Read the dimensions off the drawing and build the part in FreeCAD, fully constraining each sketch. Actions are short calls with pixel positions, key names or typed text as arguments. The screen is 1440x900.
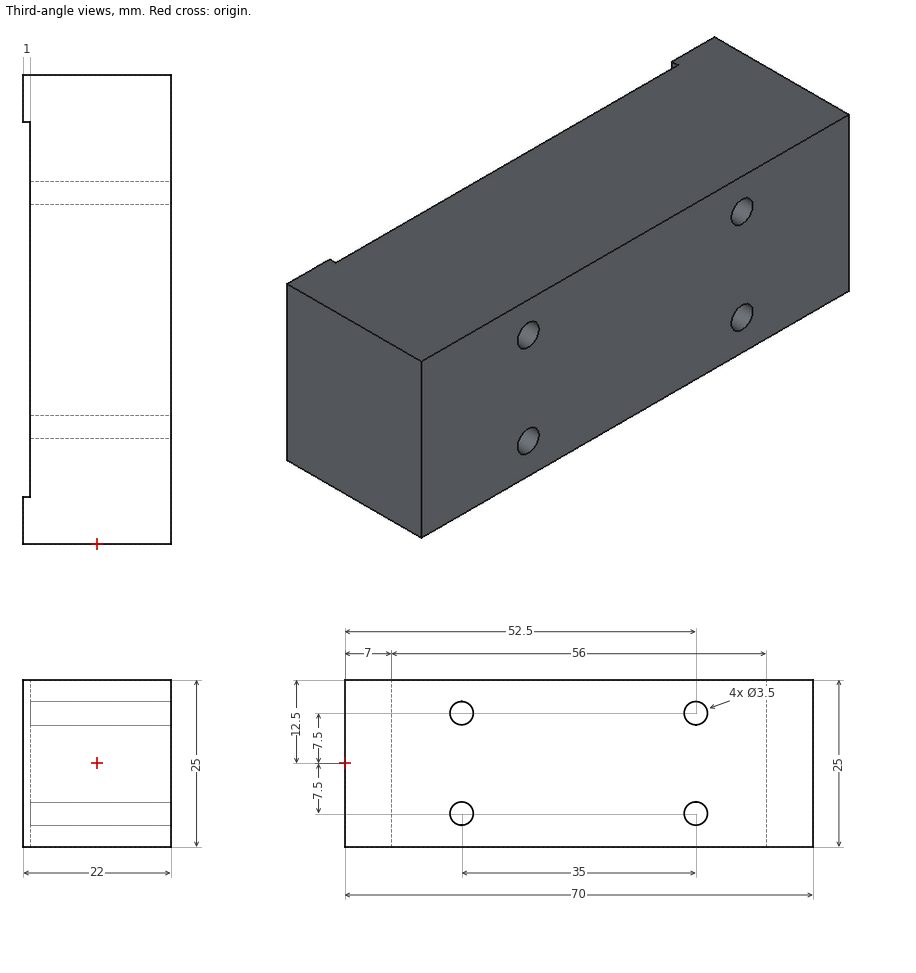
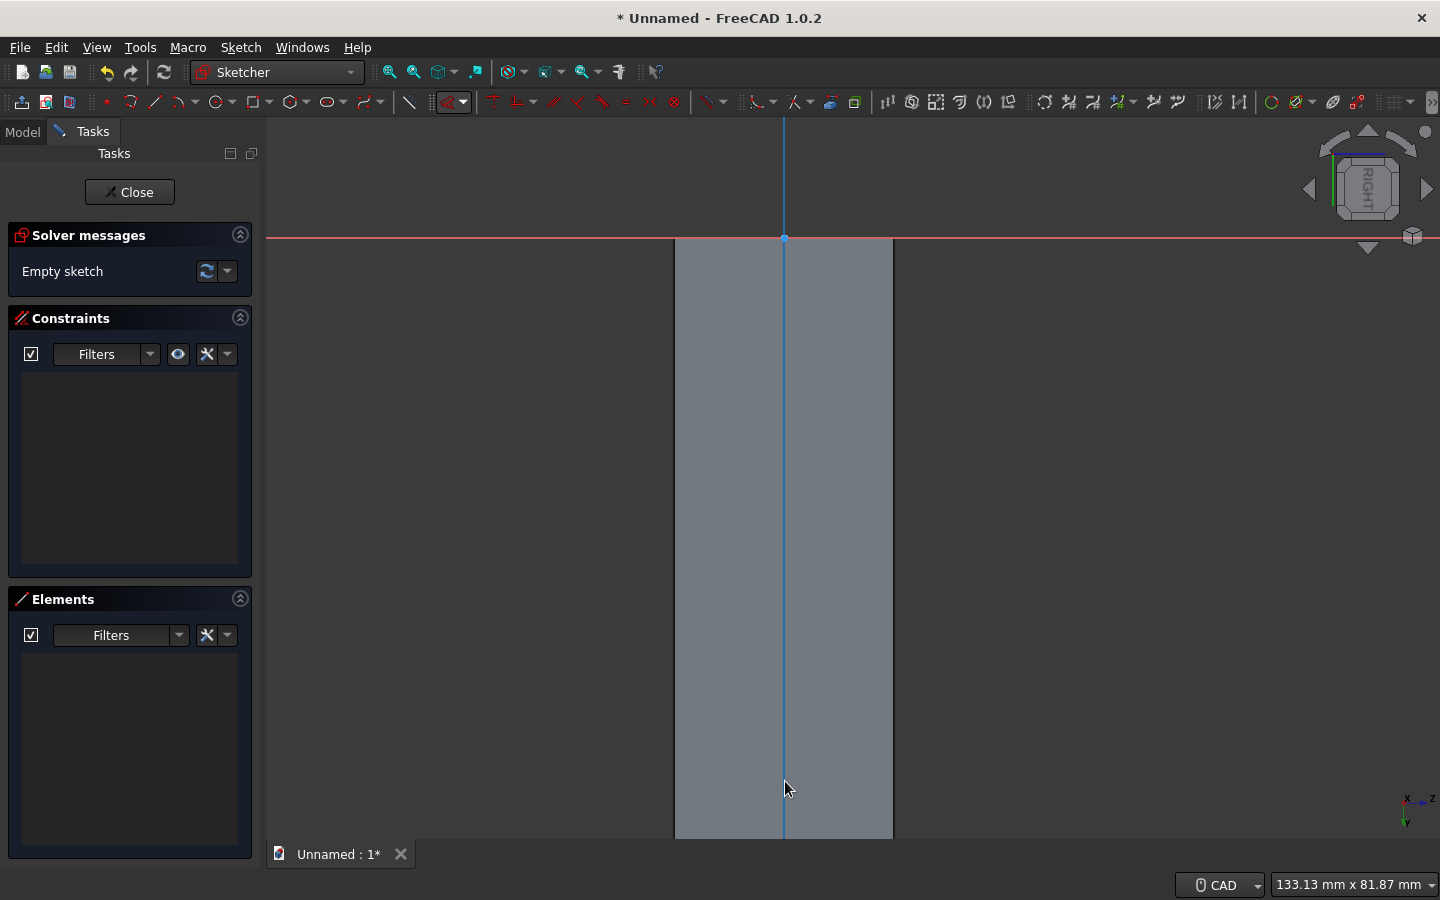
click(216, 102)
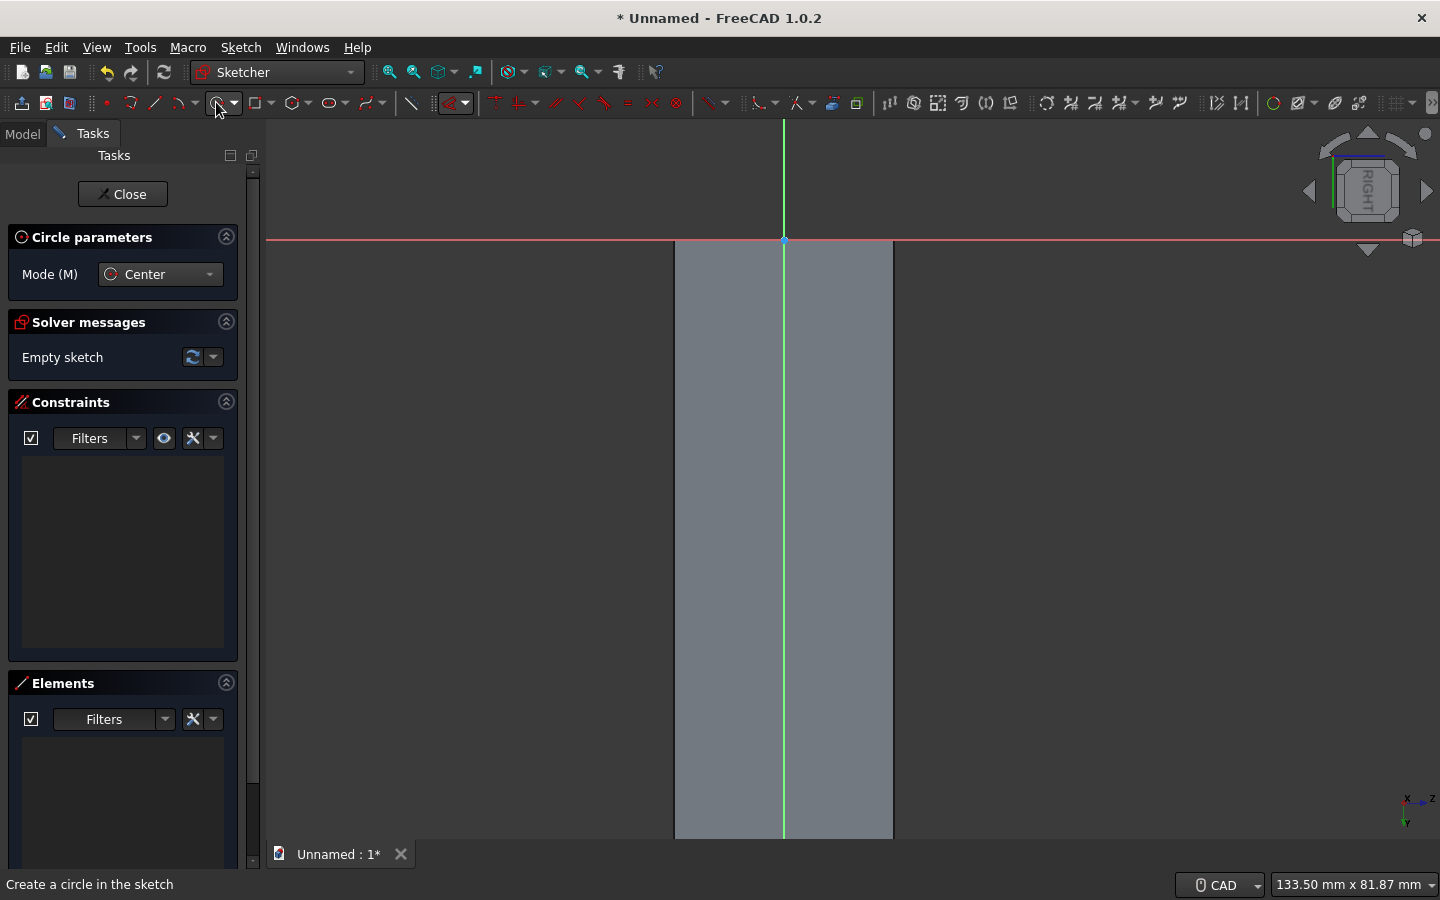
scroll(850, 702, up, 2)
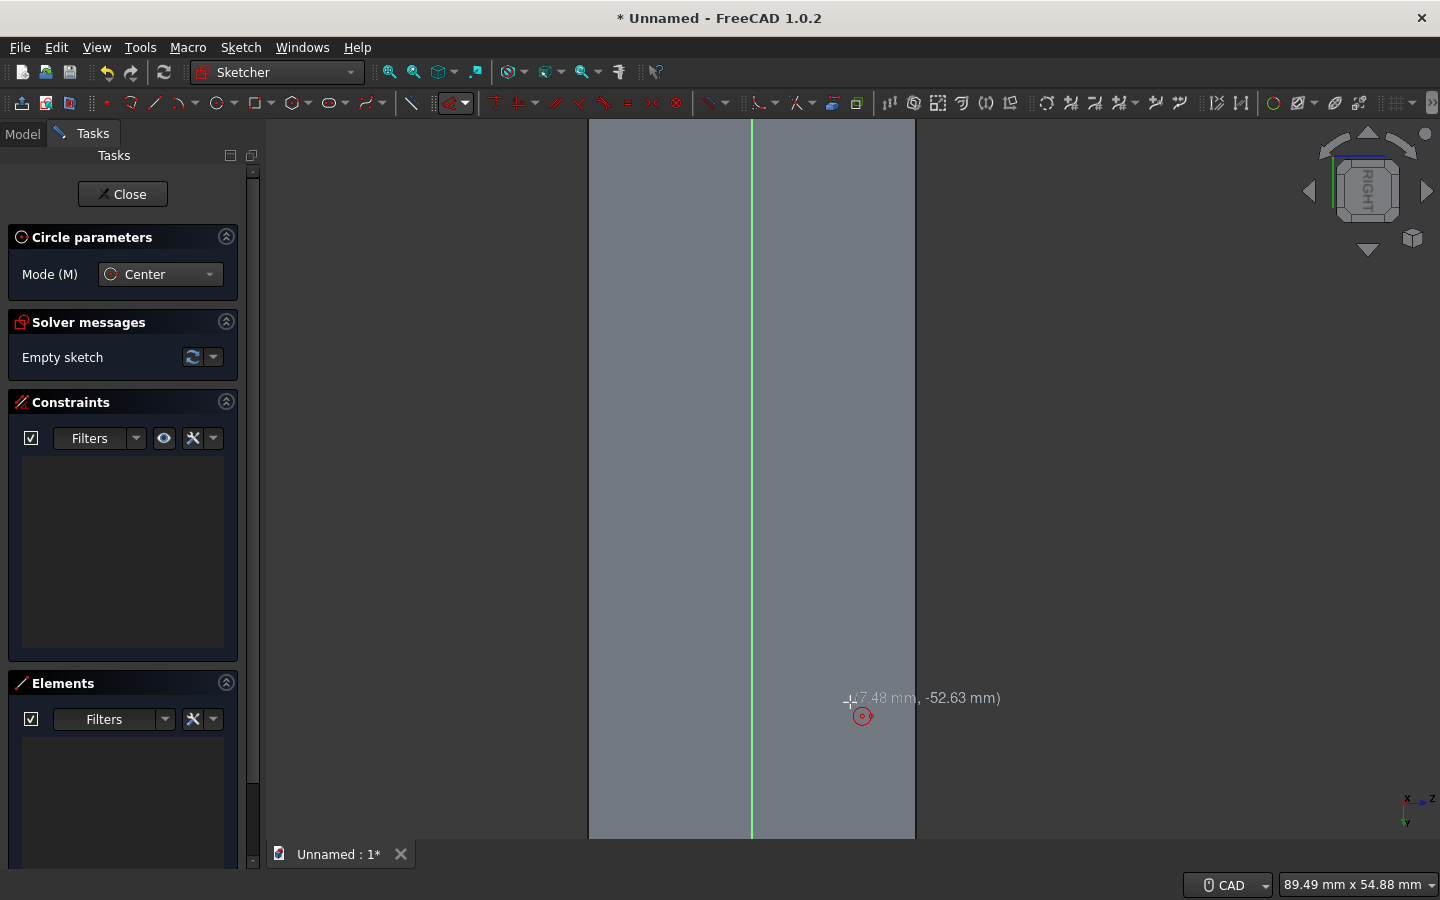
click(850, 701)
click(866, 685)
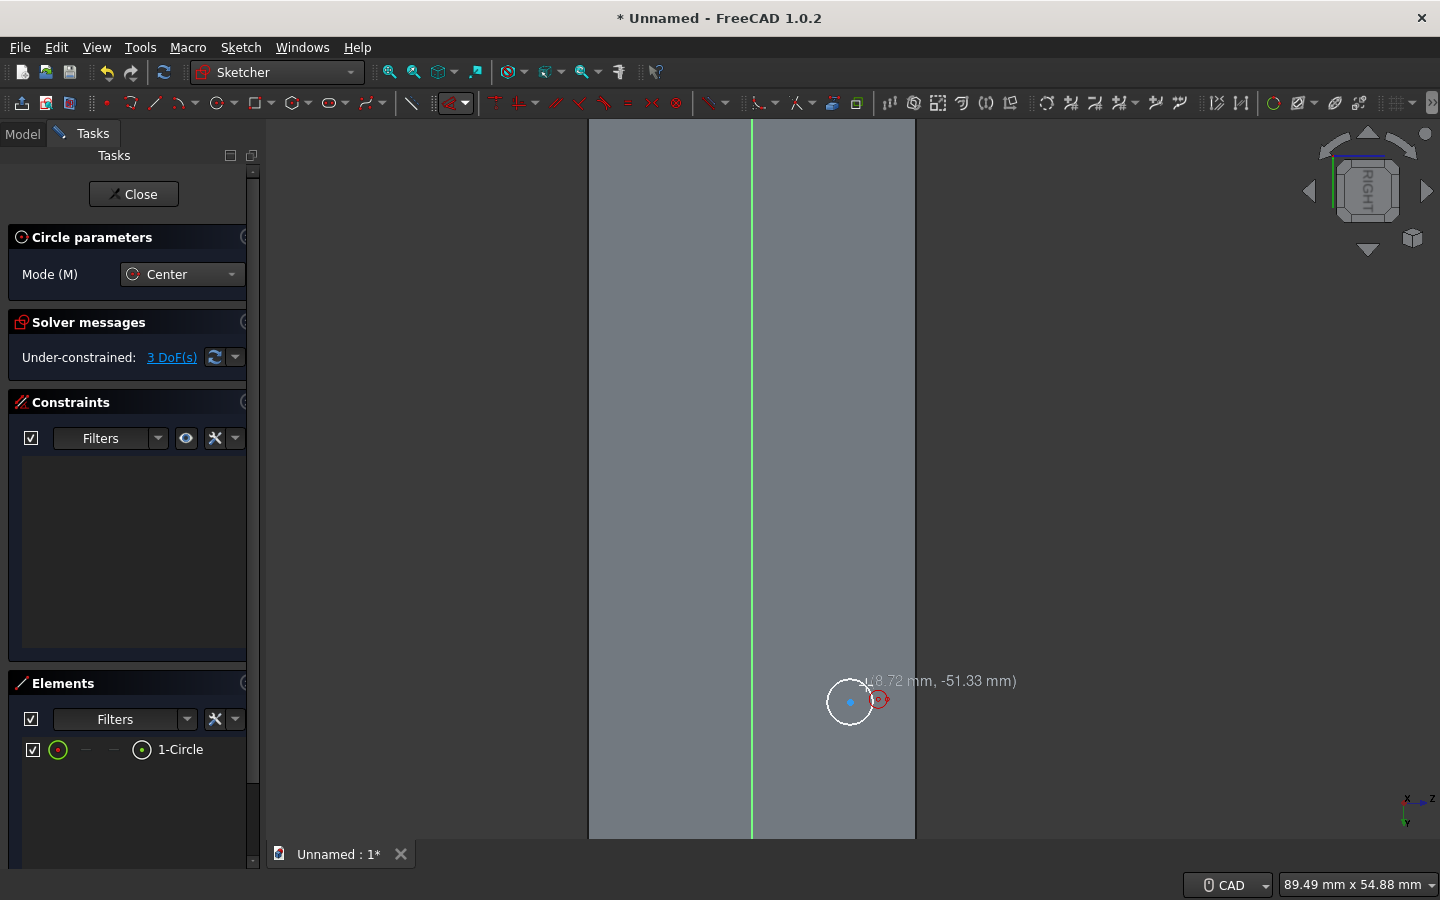
click(653, 701)
click(670, 685)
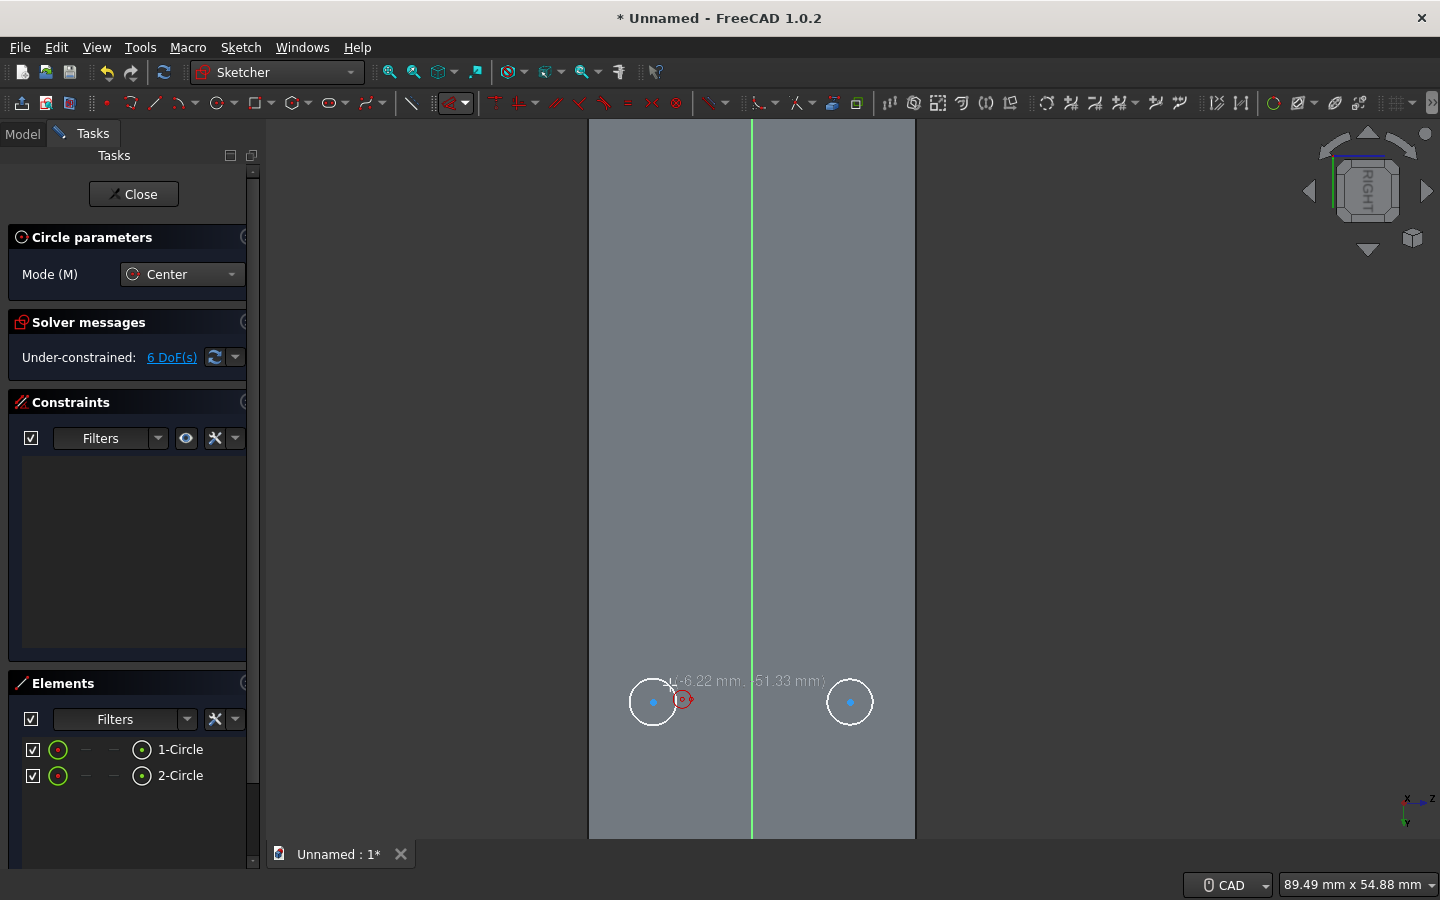
click(653, 242)
click(670, 226)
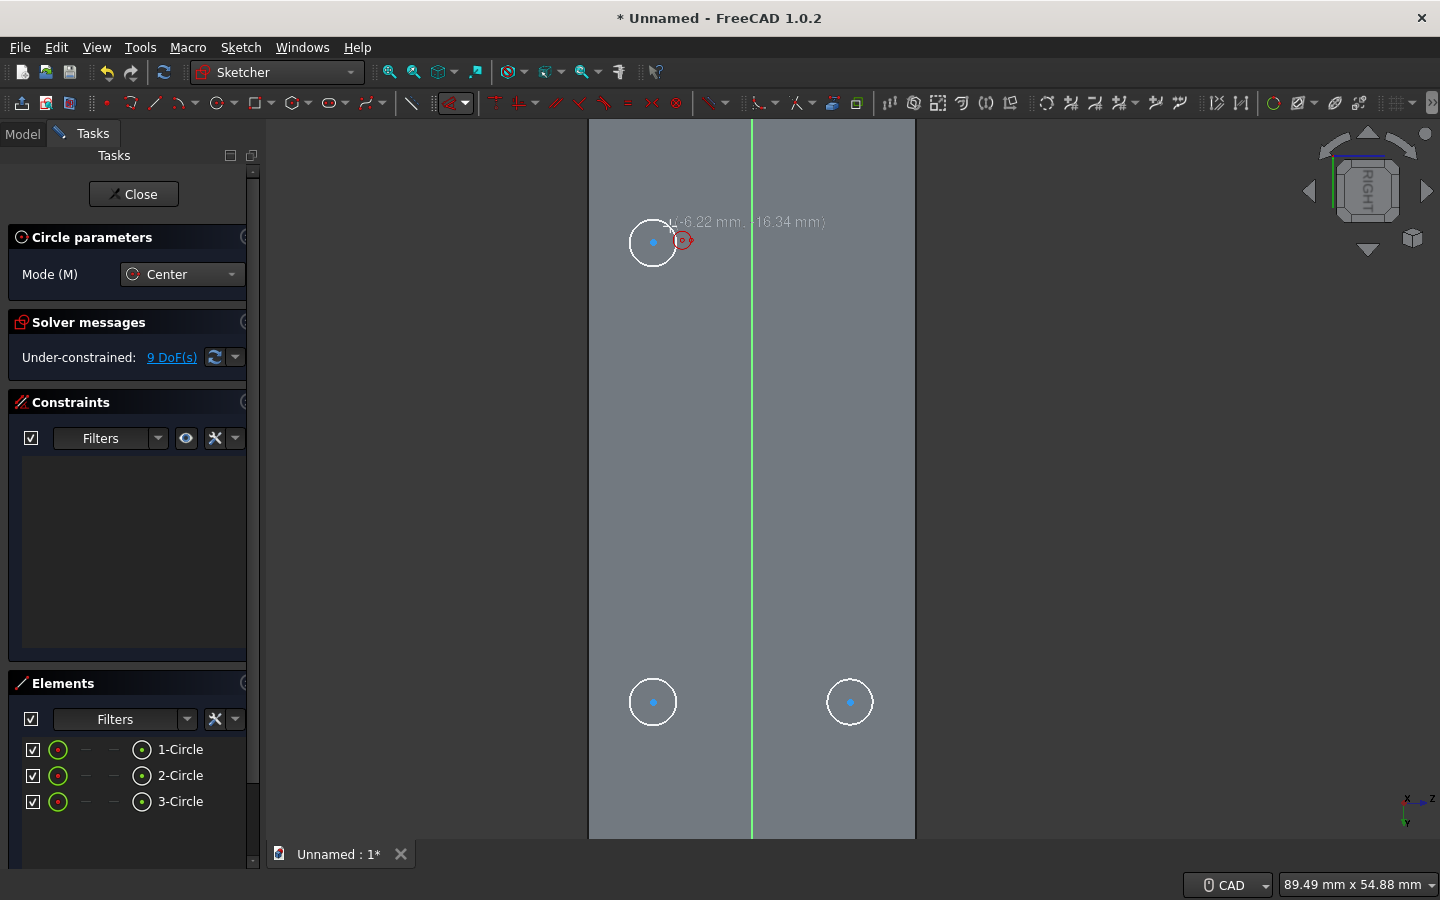
click(850, 242)
click(866, 226)
key(Escape)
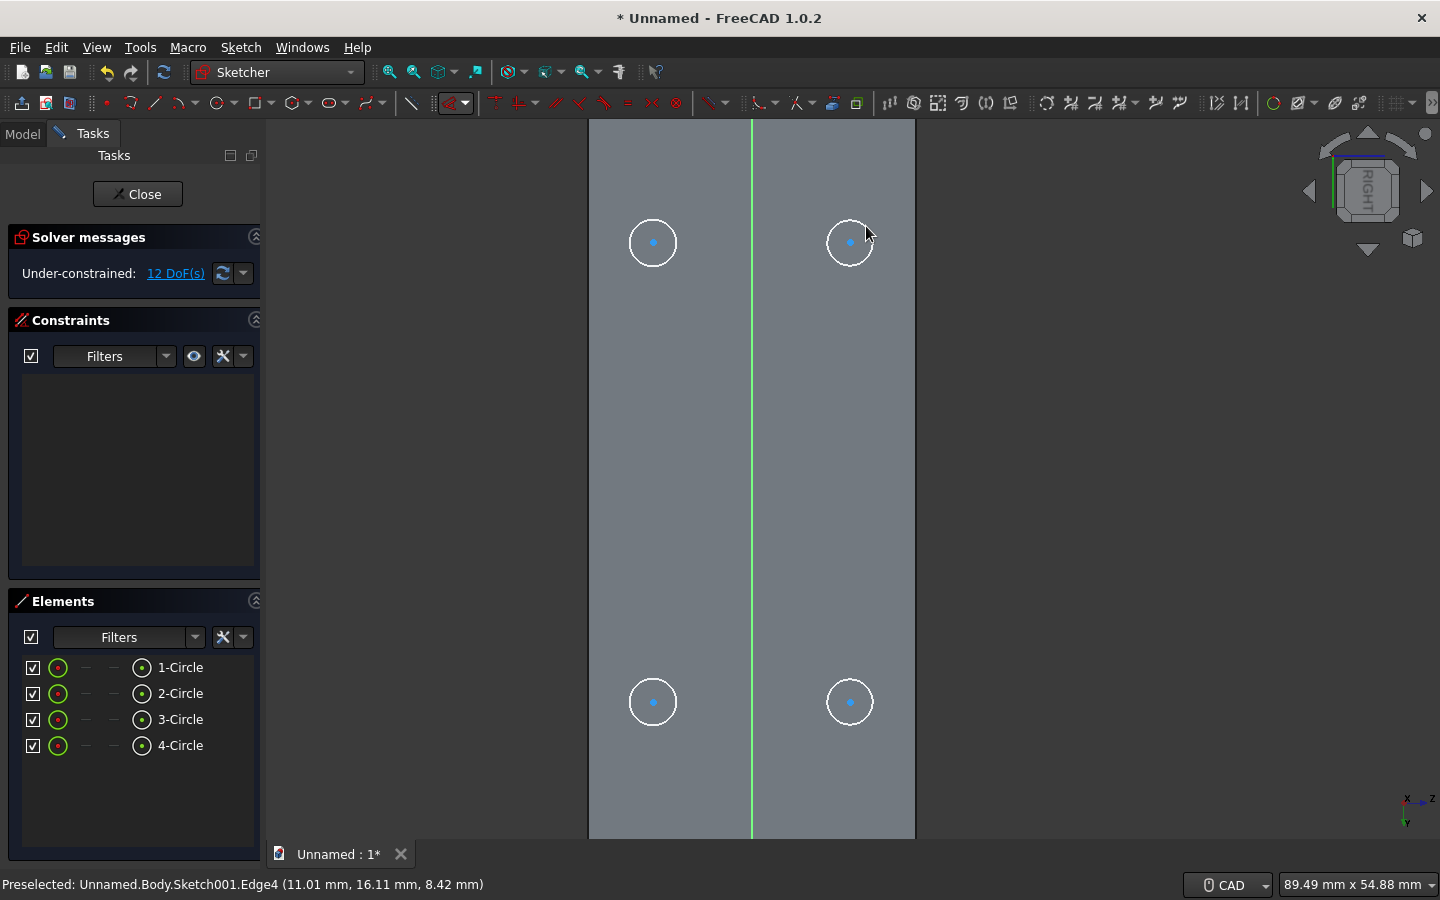
click(866, 686)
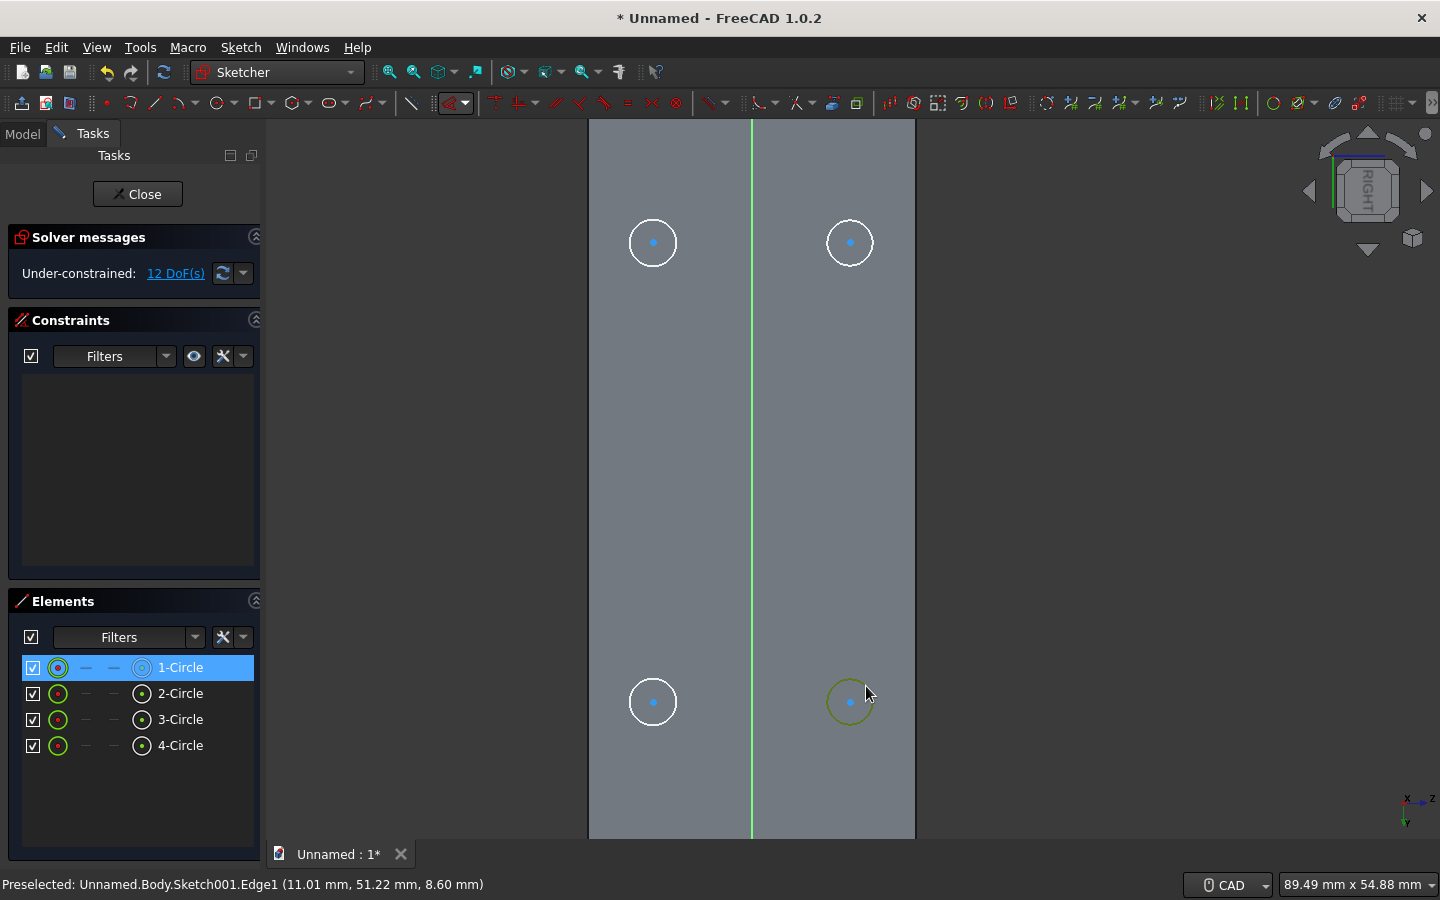
click(669, 685)